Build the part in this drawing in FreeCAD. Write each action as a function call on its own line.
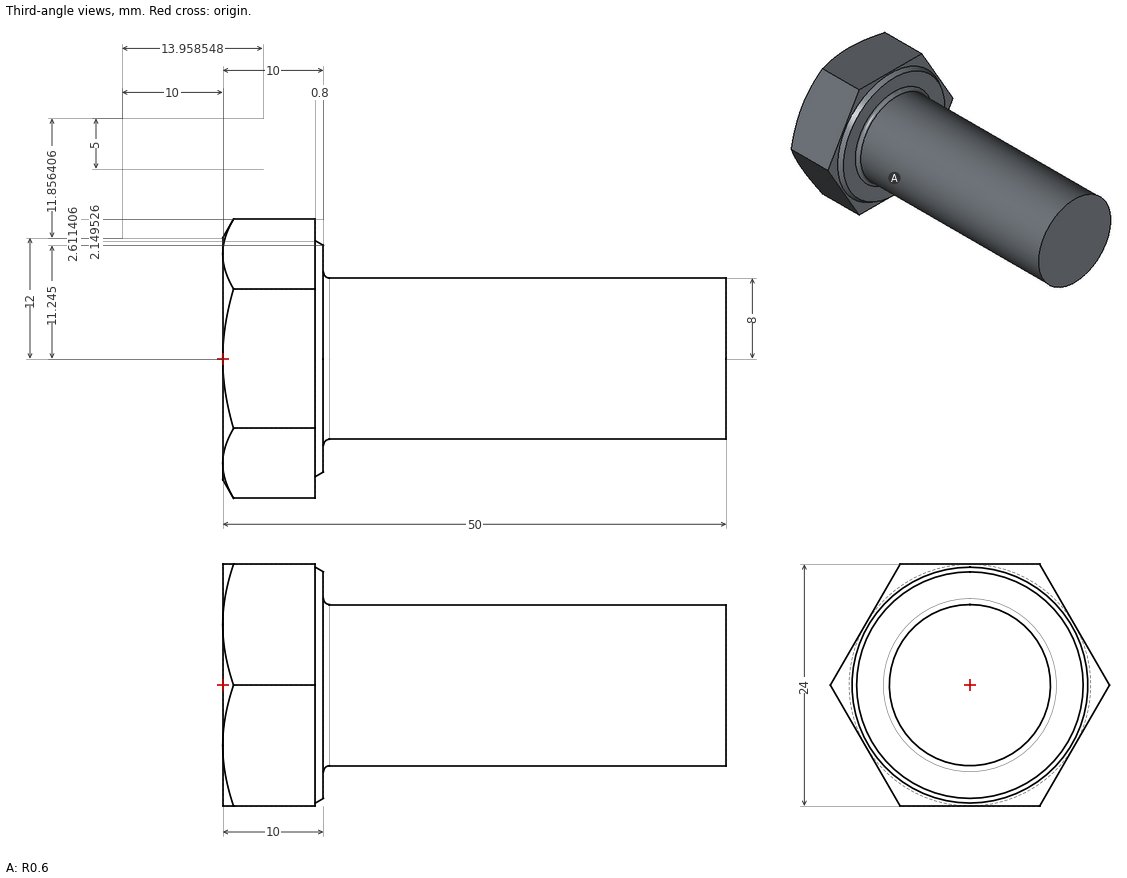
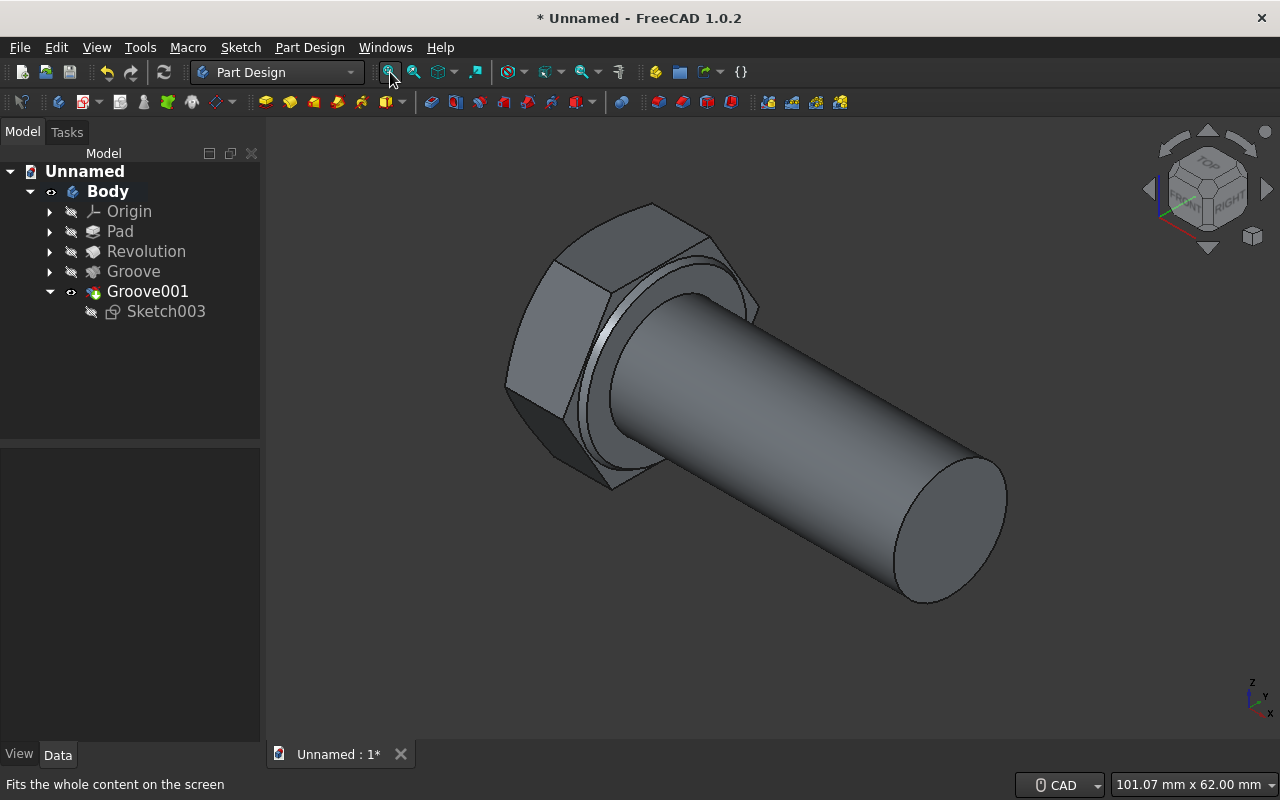
key(2)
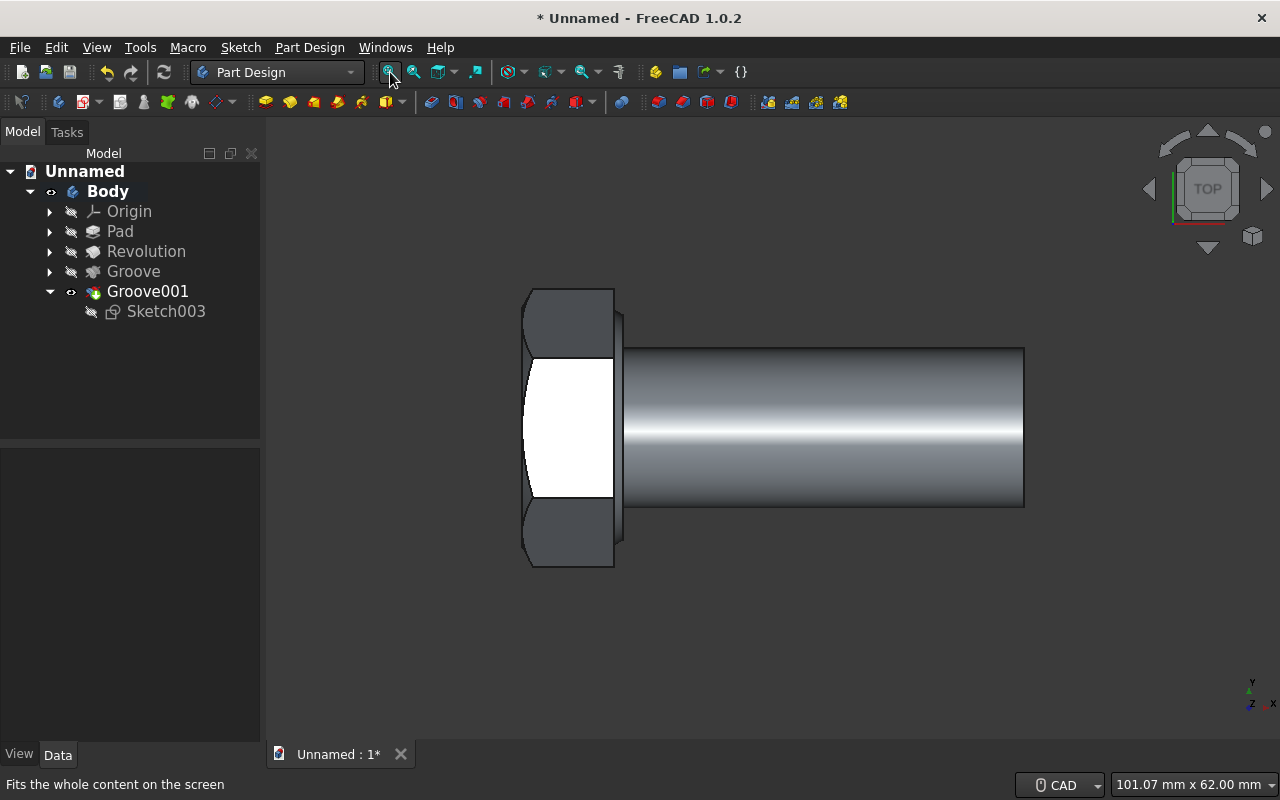
key(1)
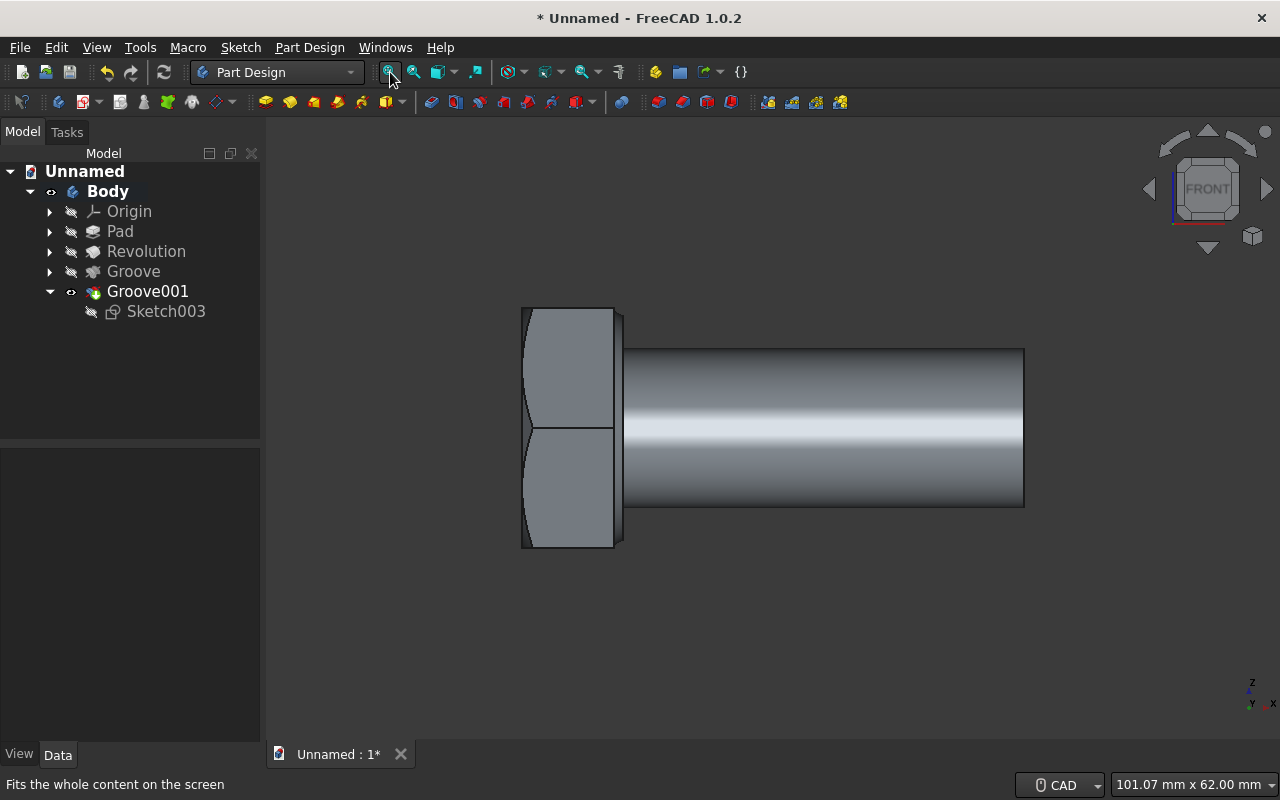
key(3)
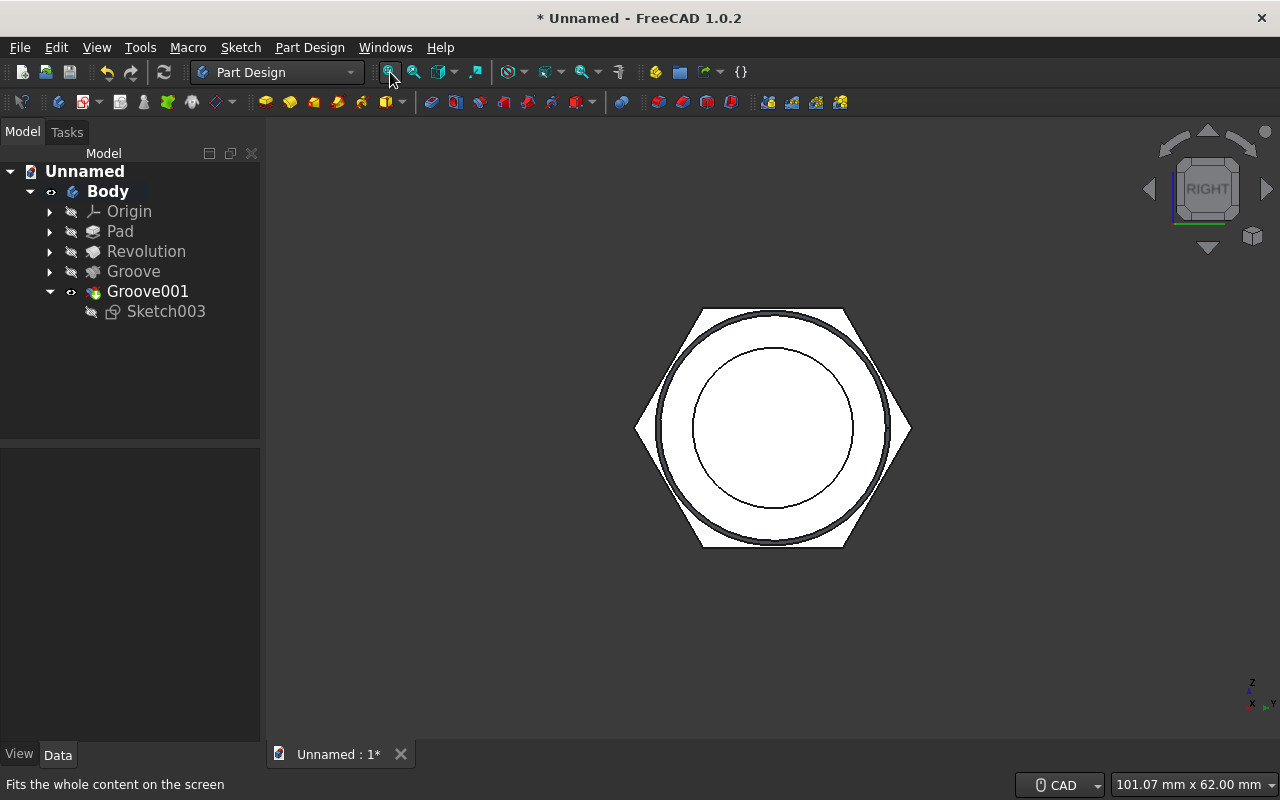
click(390, 72)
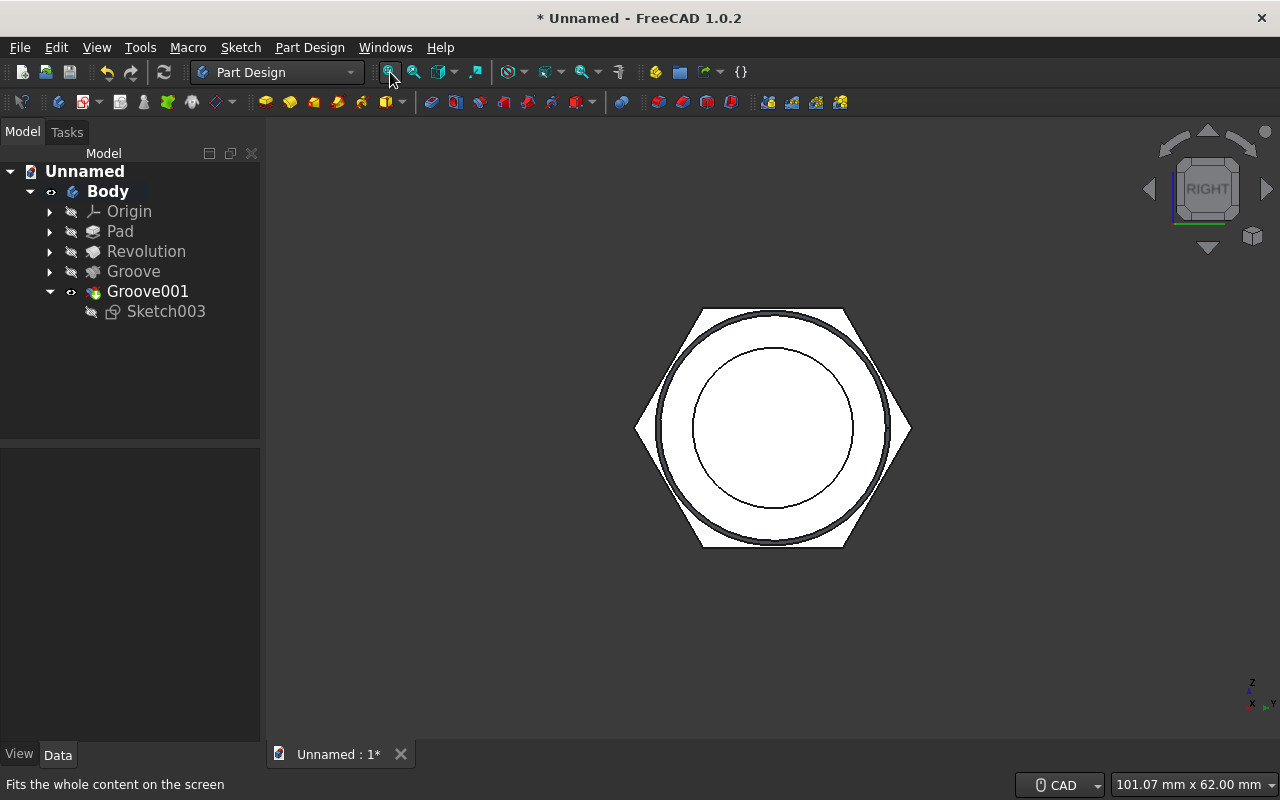
key(5)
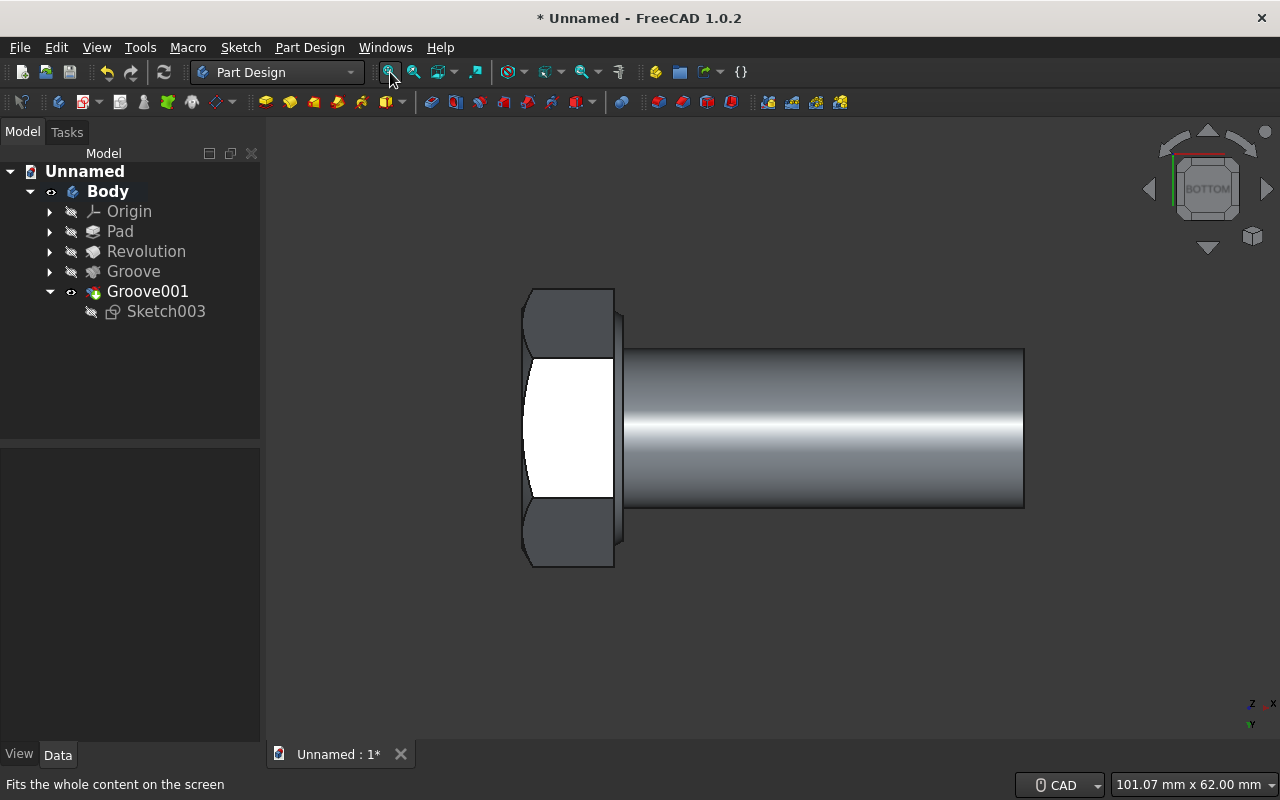
key(4)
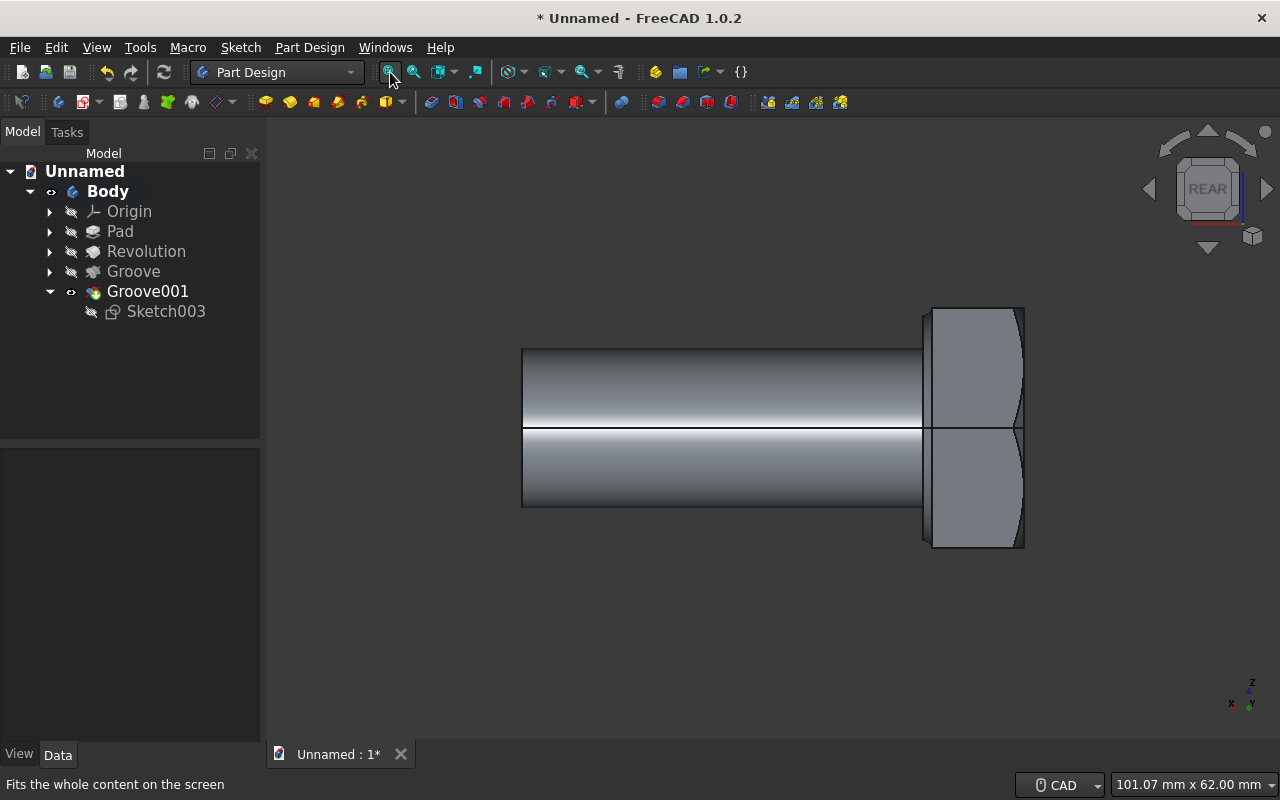
key(6)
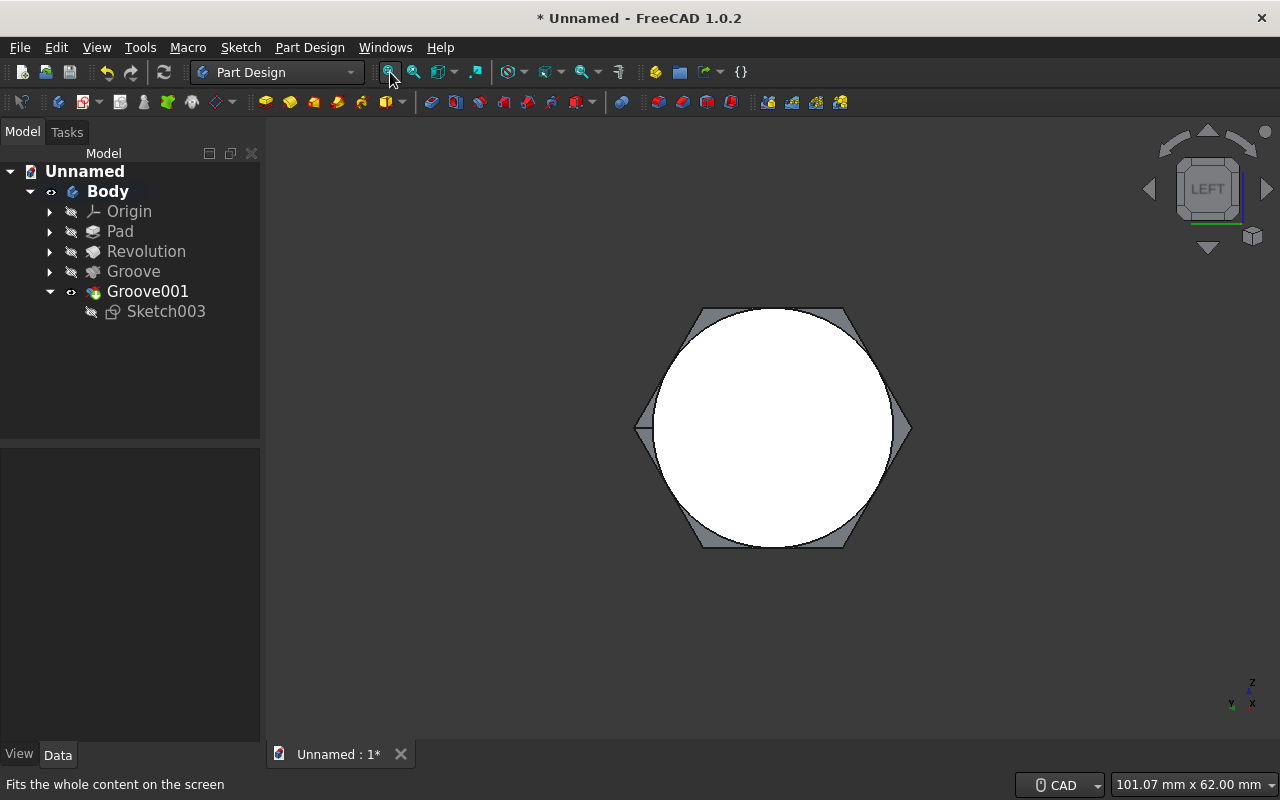
click(390, 72)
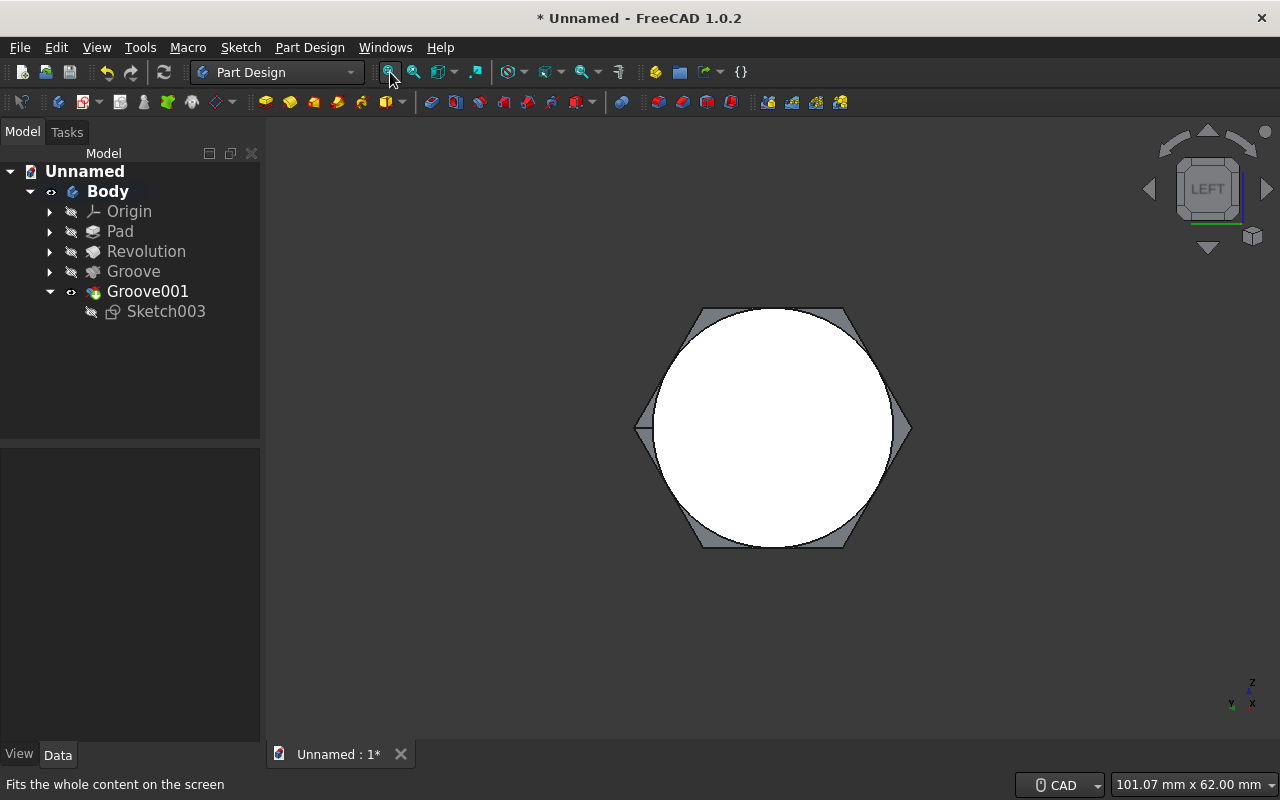
key(v)
key(3)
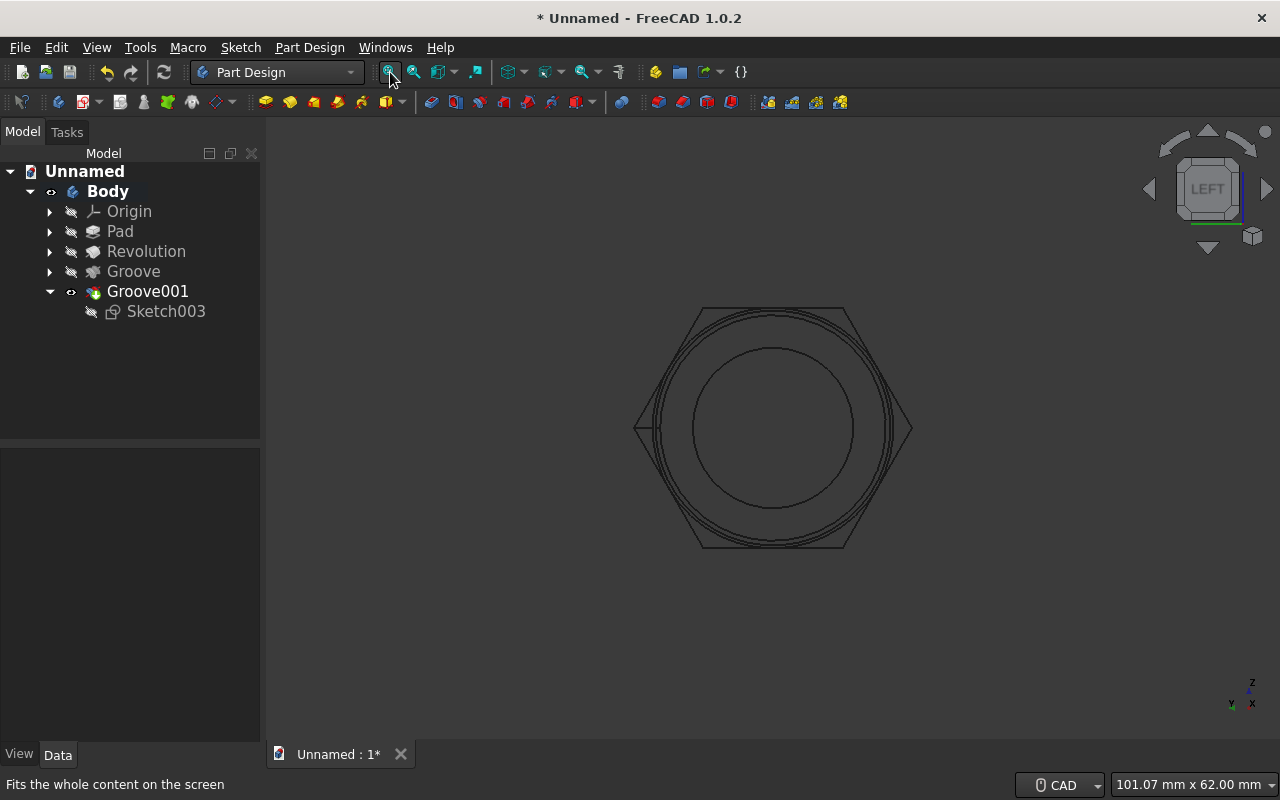
key(0)